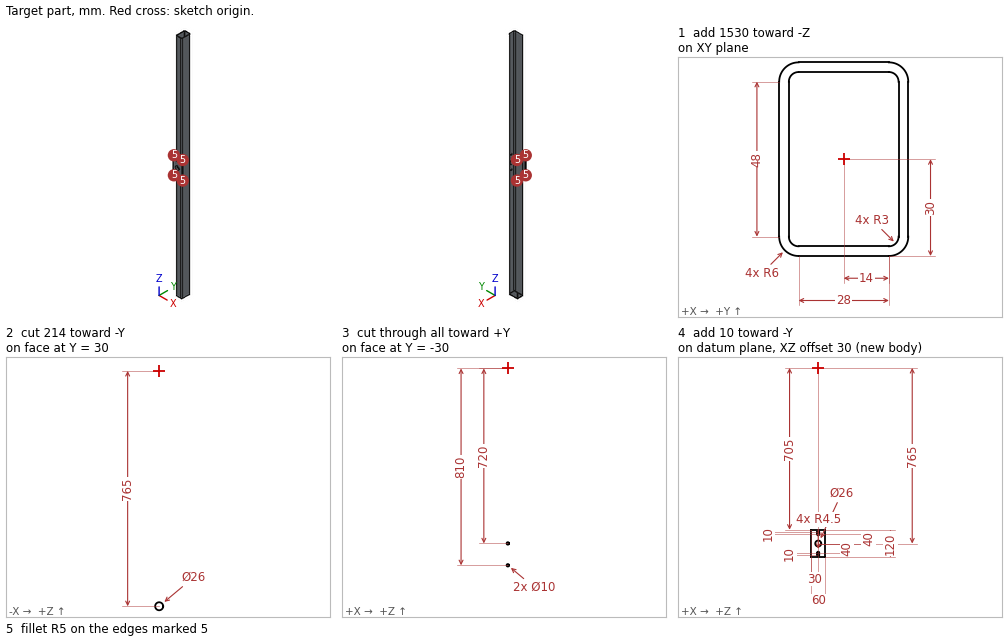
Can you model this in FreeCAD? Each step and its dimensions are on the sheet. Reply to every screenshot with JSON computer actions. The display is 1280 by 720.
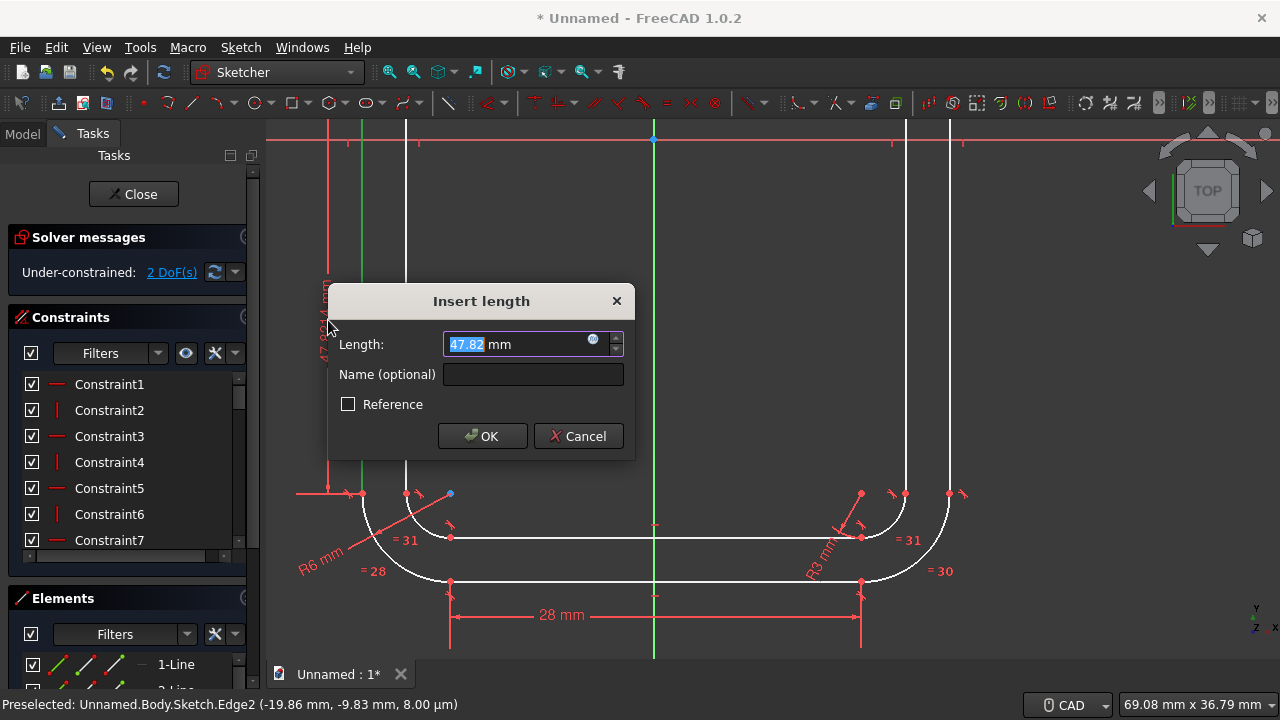
{"action": "type", "text": "48"}
{"action": "key", "text": "Return"}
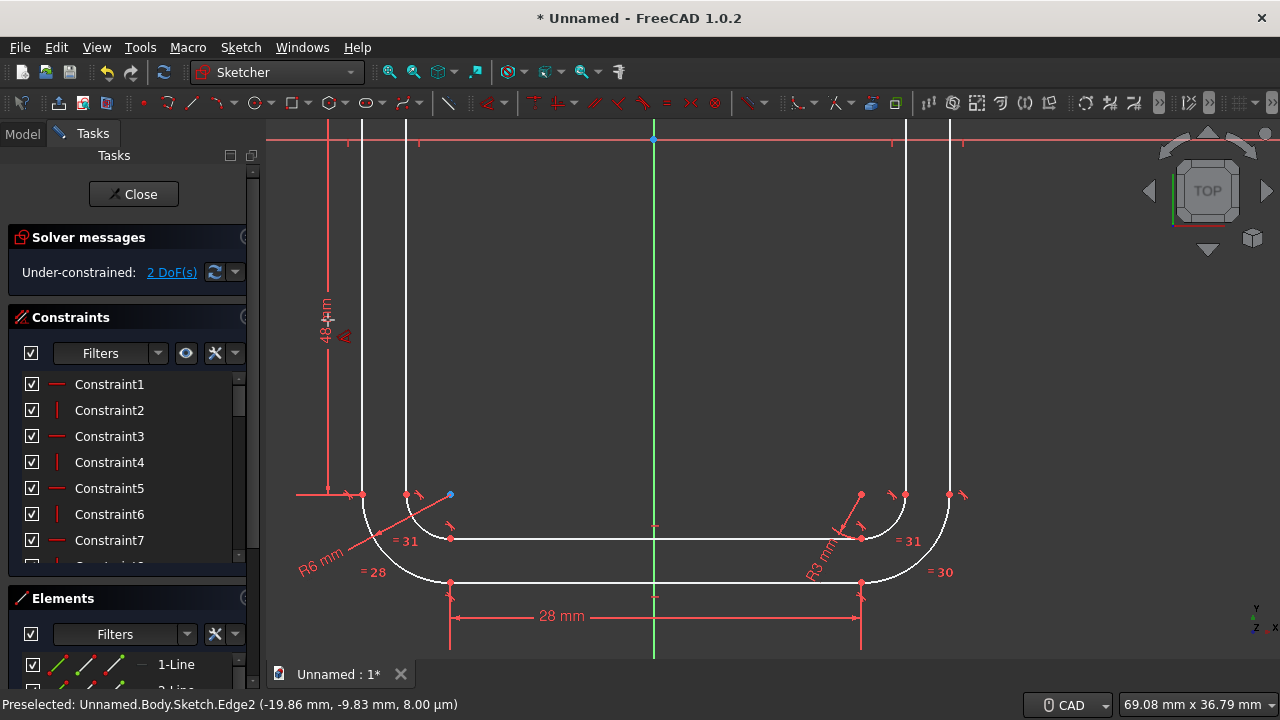
{"action": "left_click", "coordinate": [862, 583]}
{"action": "left_click", "coordinate": [758, 617]}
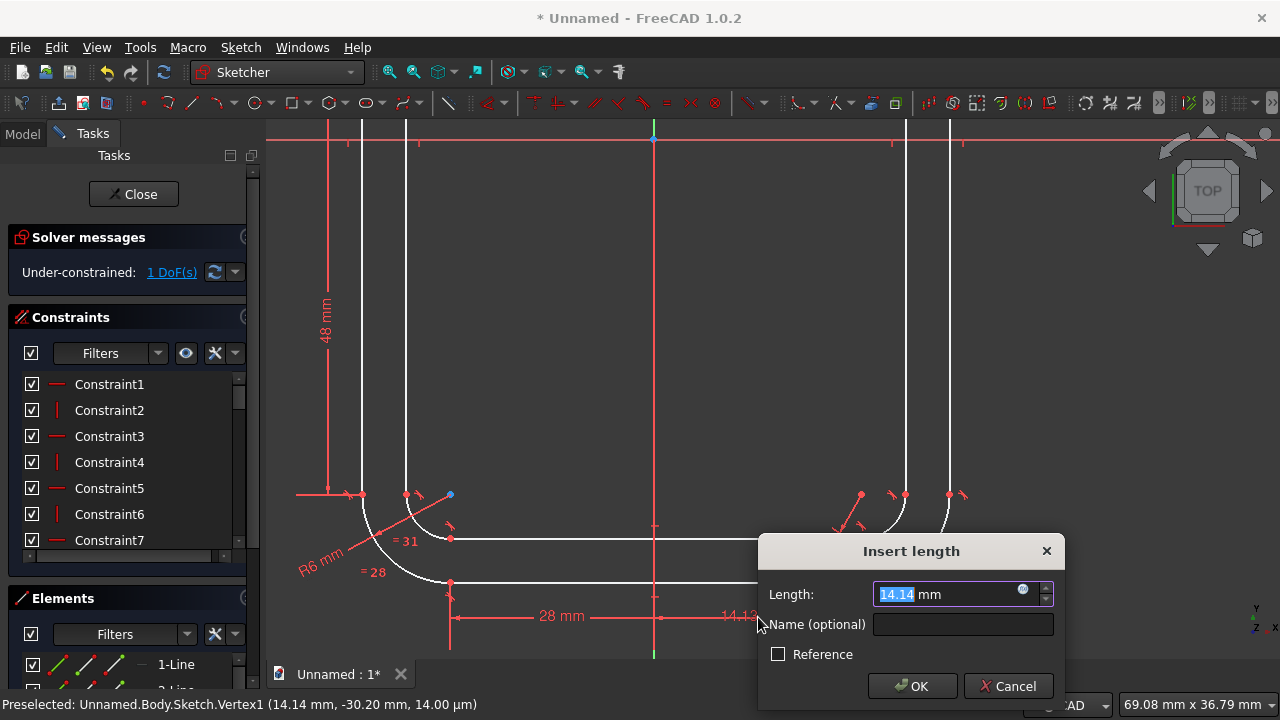
{"action": "type", "text": "14"}
{"action": "key", "text": "Return"}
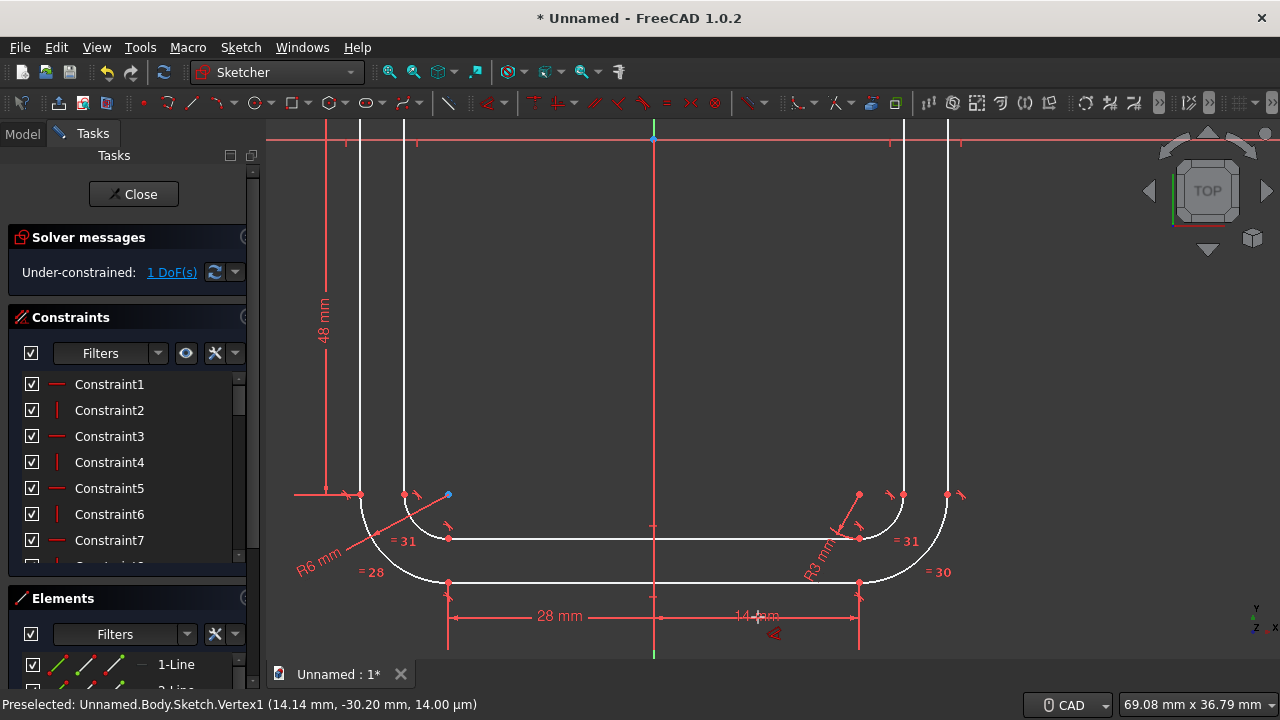
{"action": "left_click", "coordinate": [859, 583]}
{"action": "left_click", "coordinate": [620, 365]}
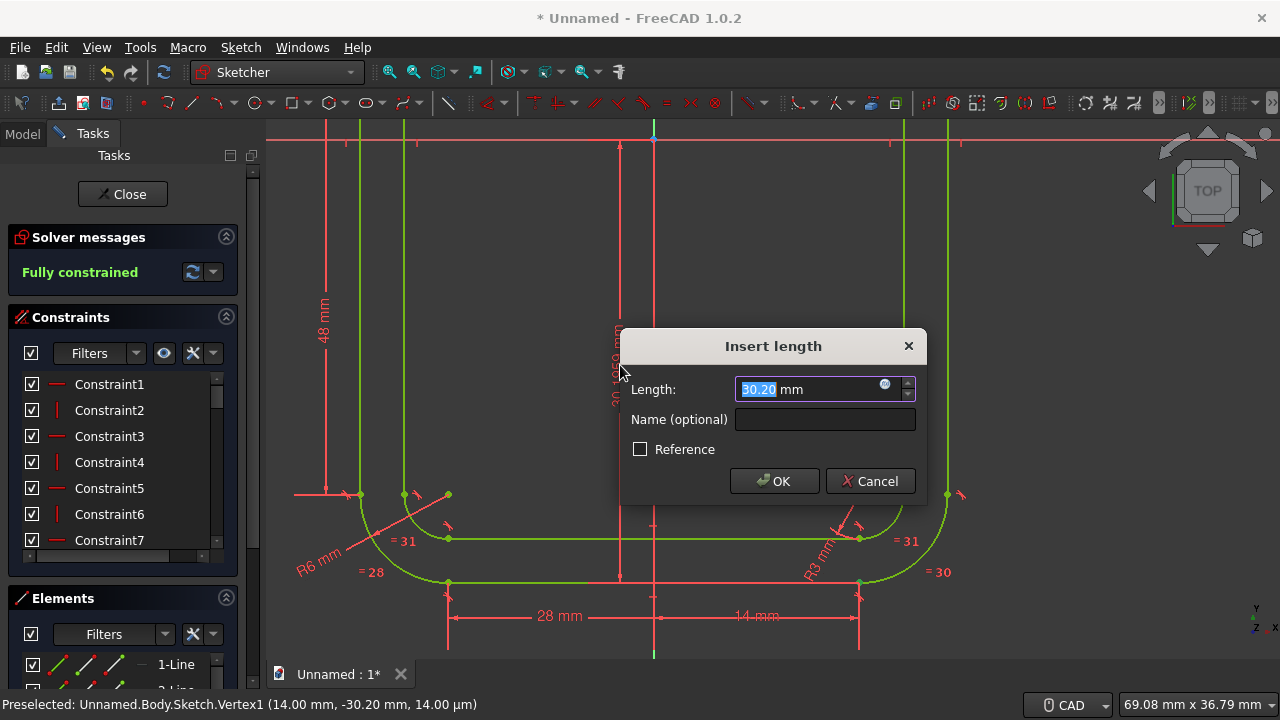
{"action": "type", "text": "30"}
{"action": "key", "text": "Return"}
{"action": "key", "text": "Escape"}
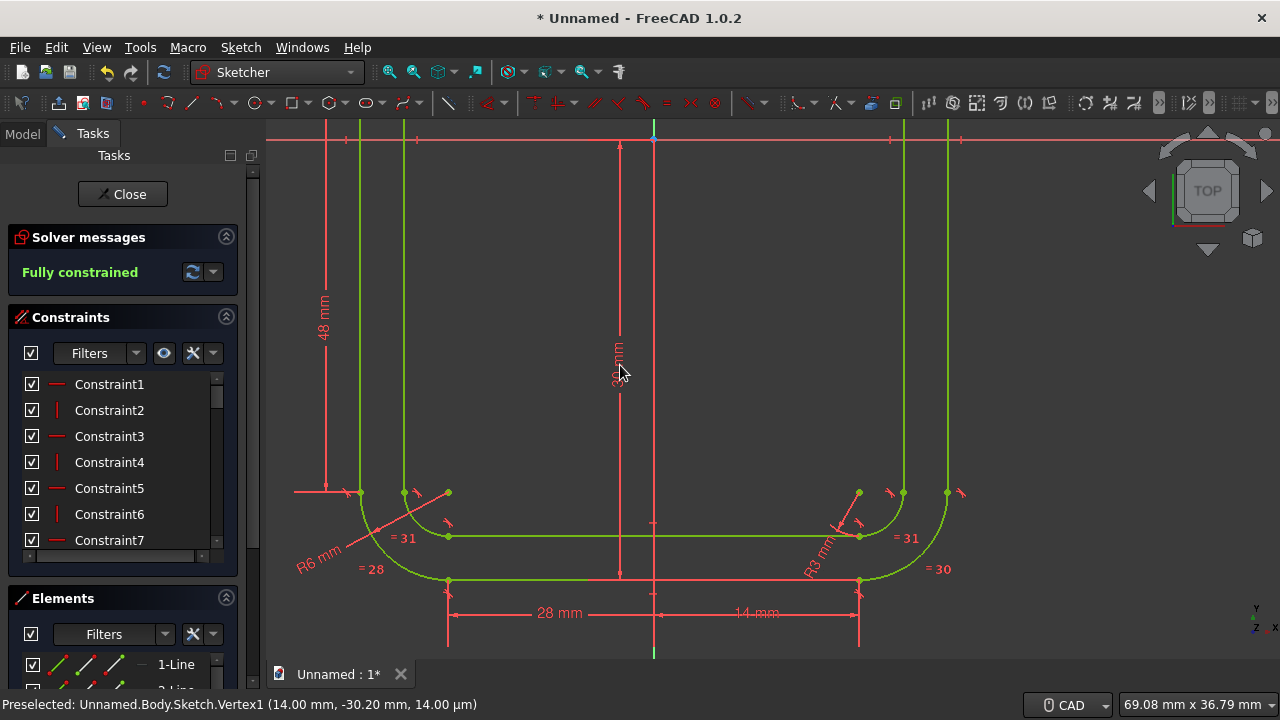
{"action": "left_click", "coordinate": [123, 194]}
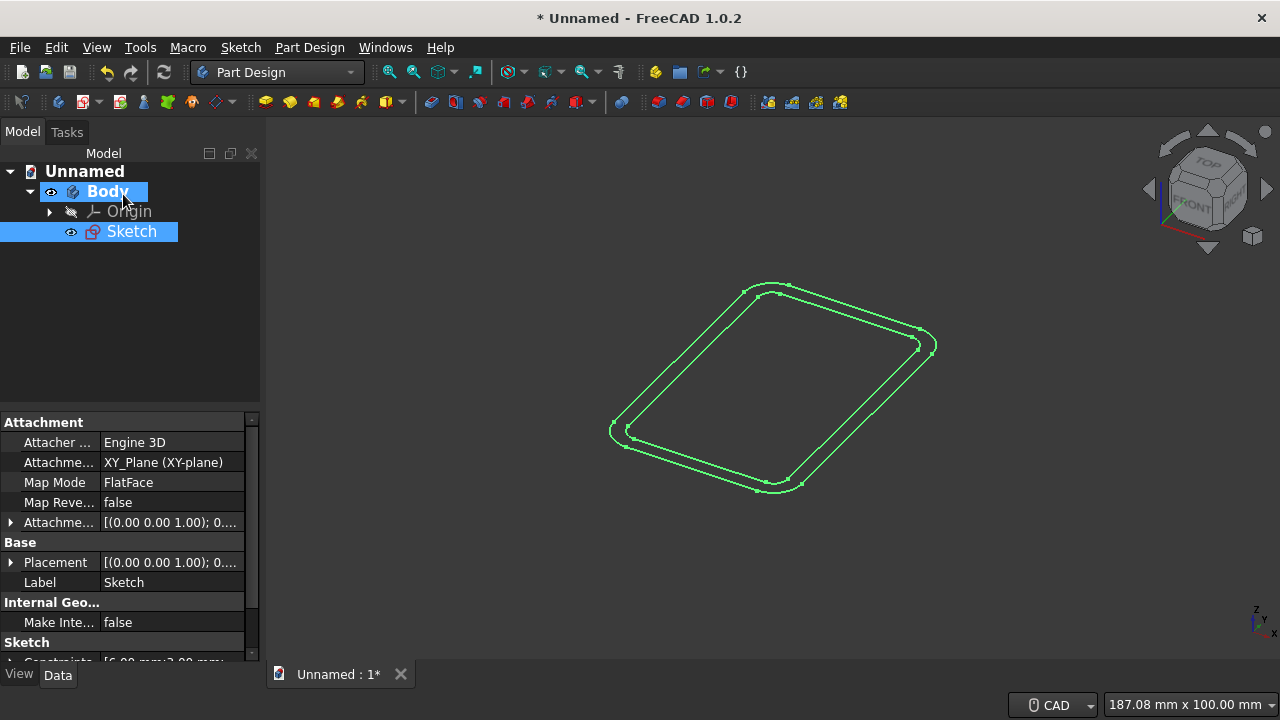
{"action": "left_click", "coordinate": [266, 102]}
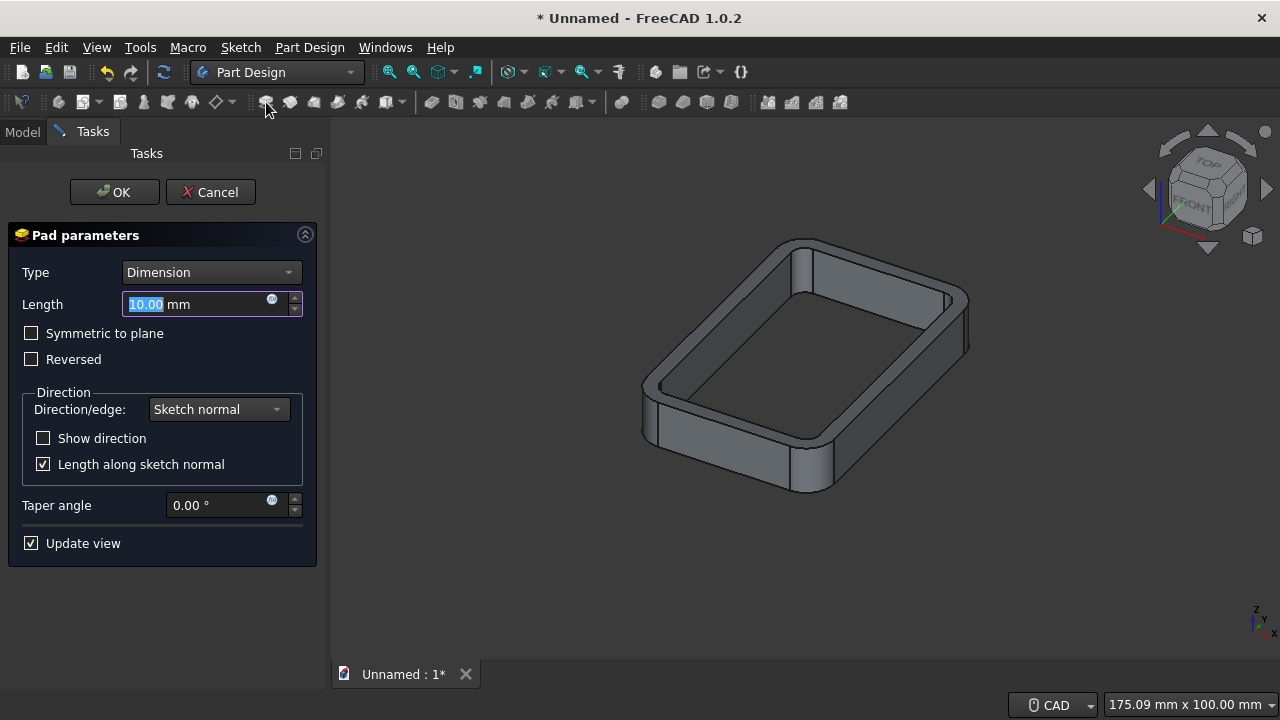
{"action": "type", "text": "1530"}
{"action": "key", "text": "Tab"}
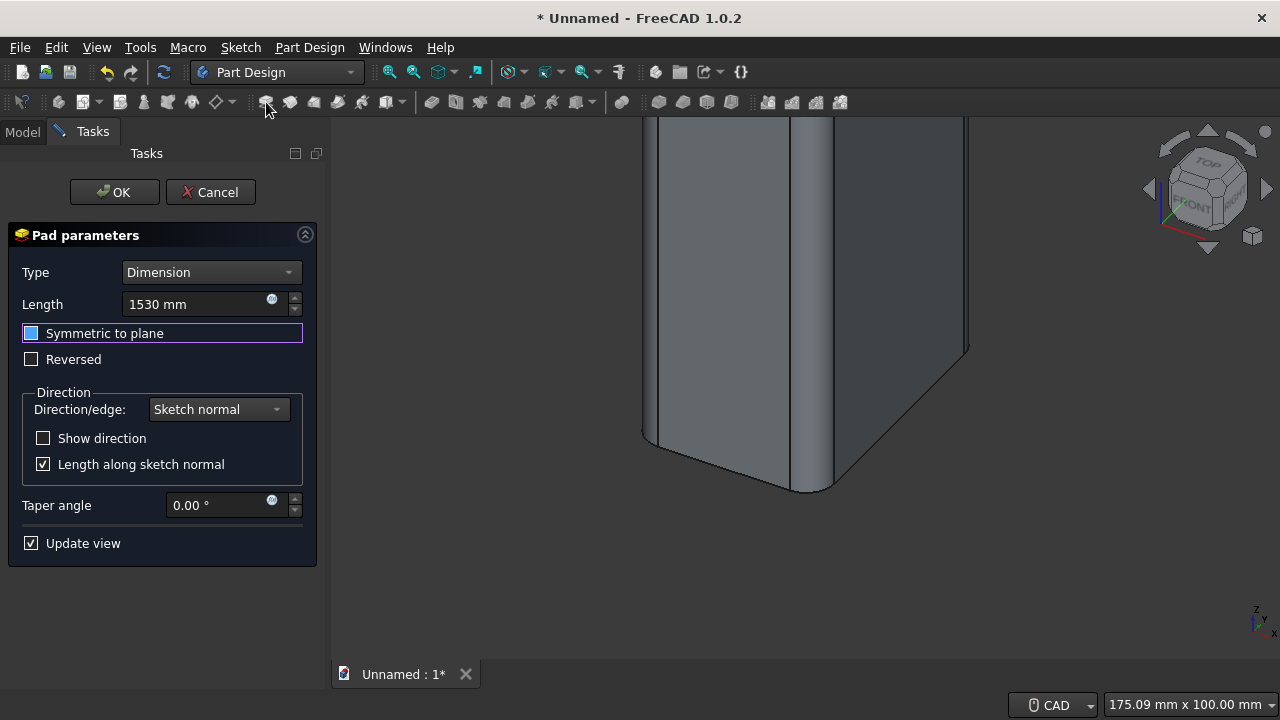
{"action": "left_click", "coordinate": [30, 359]}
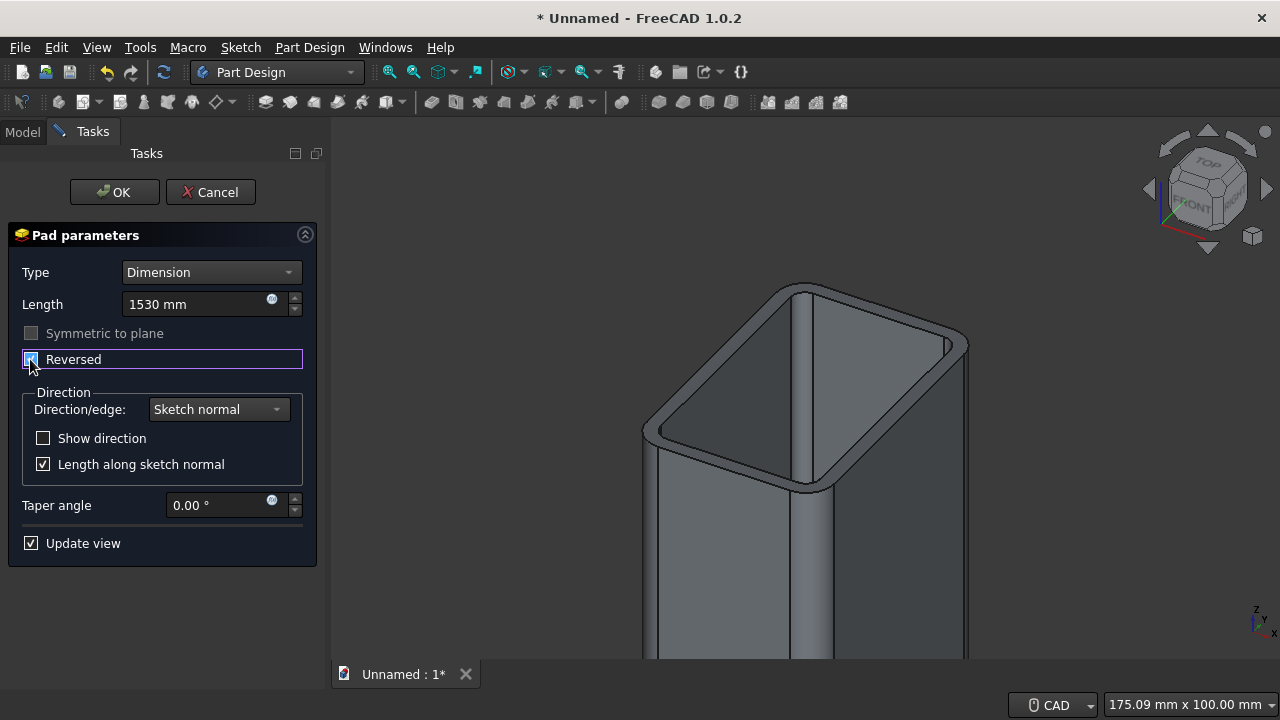
{"action": "left_click", "coordinate": [115, 192]}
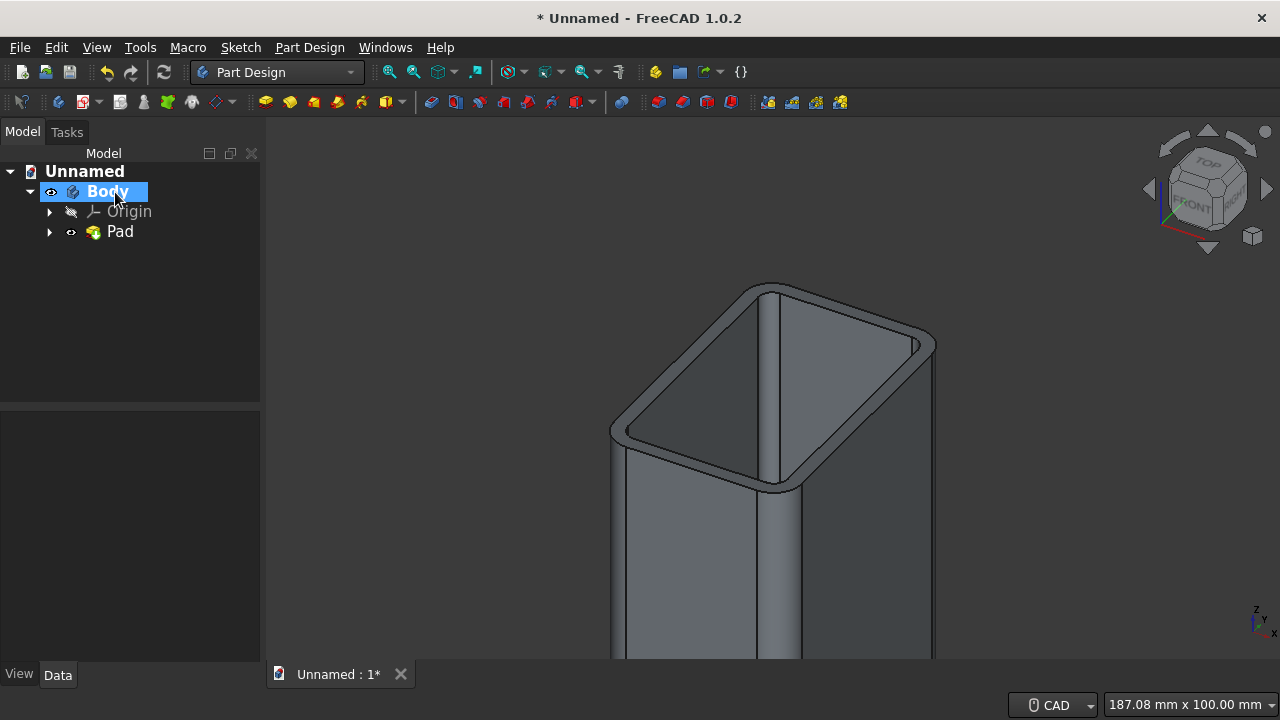
{"action": "left_click", "coordinate": [390, 72]}